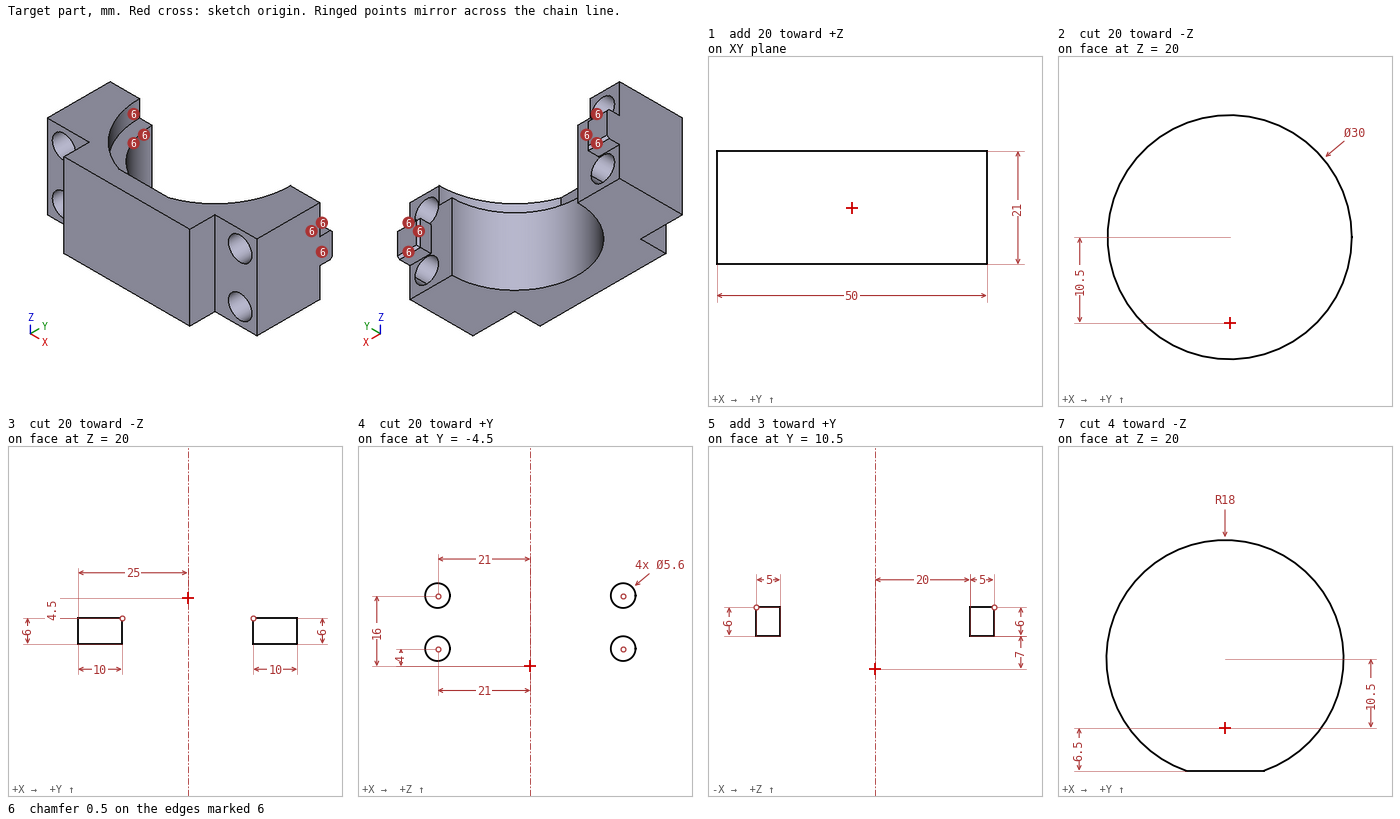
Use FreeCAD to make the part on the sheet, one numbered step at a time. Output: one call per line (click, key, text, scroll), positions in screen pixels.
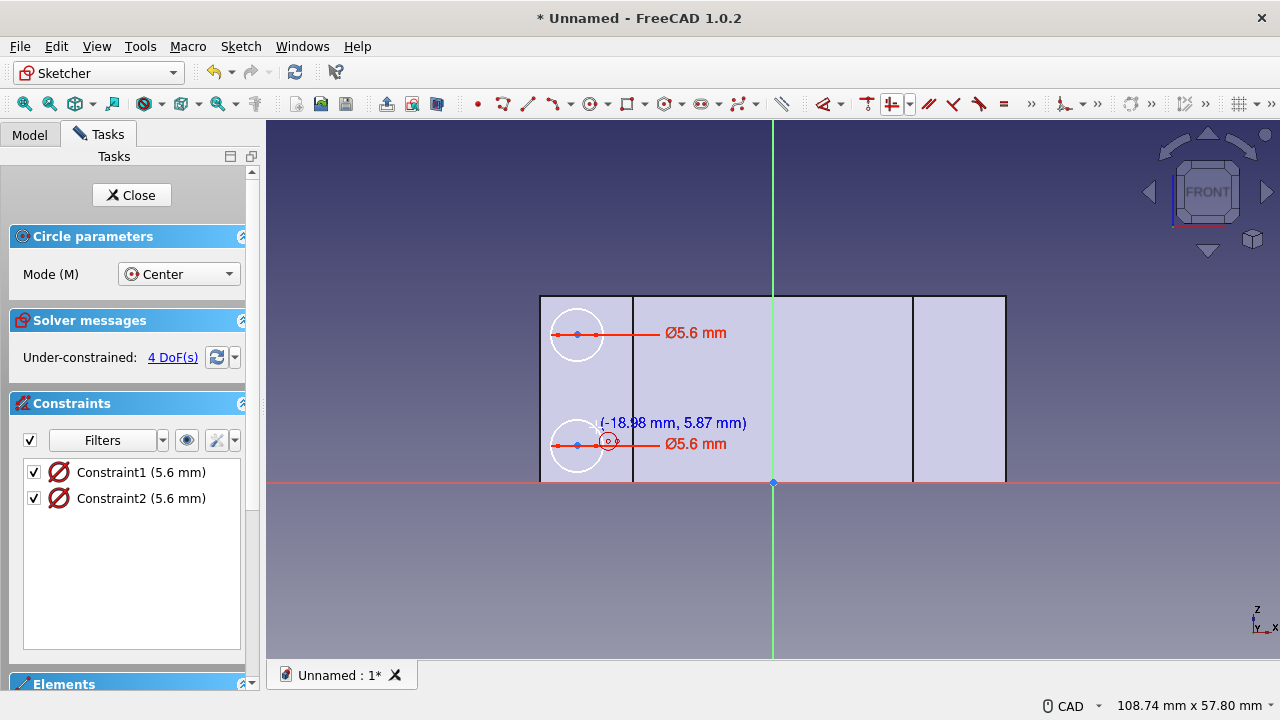
click(969, 334)
move(987, 315)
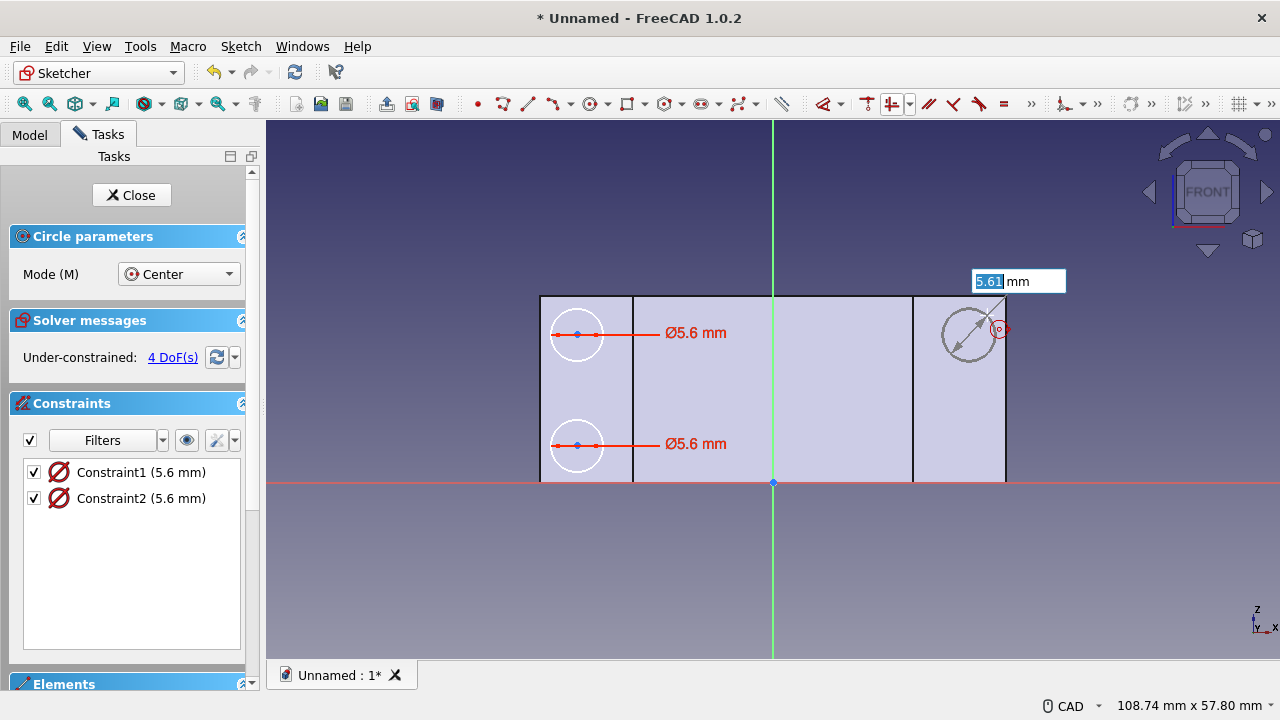
text(5.6)
key(Return)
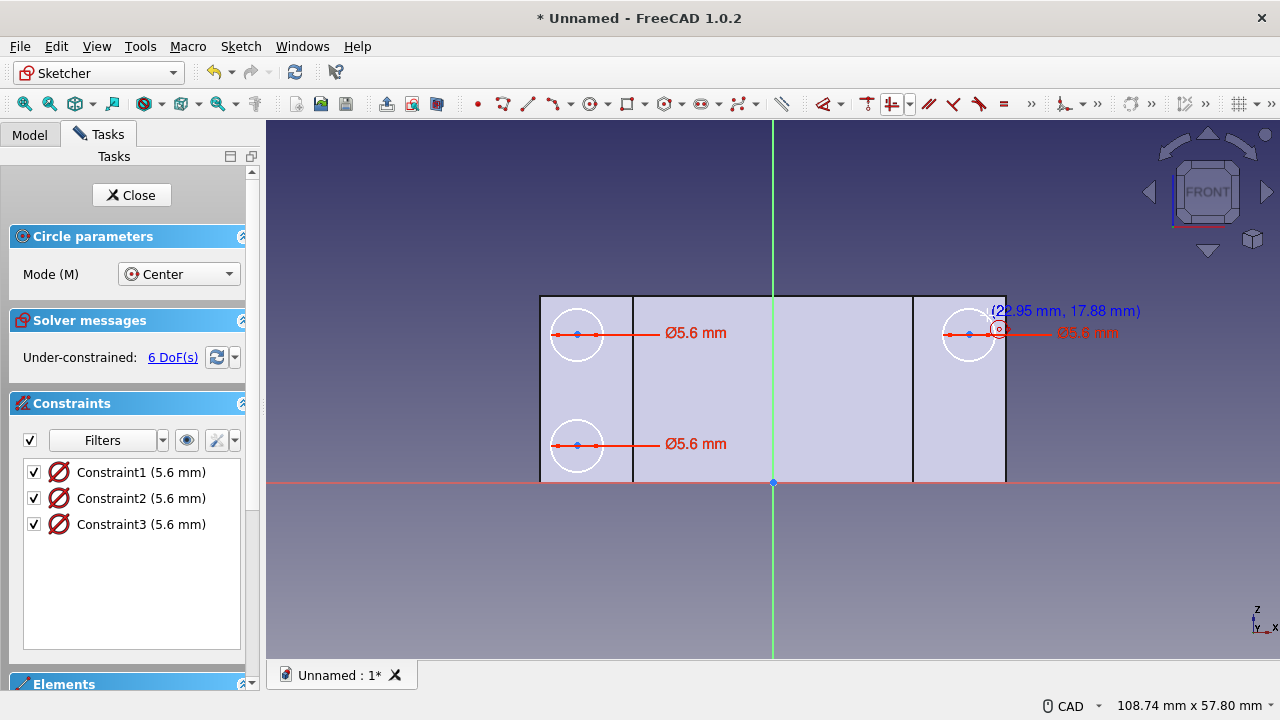
click(969, 445)
move(987, 427)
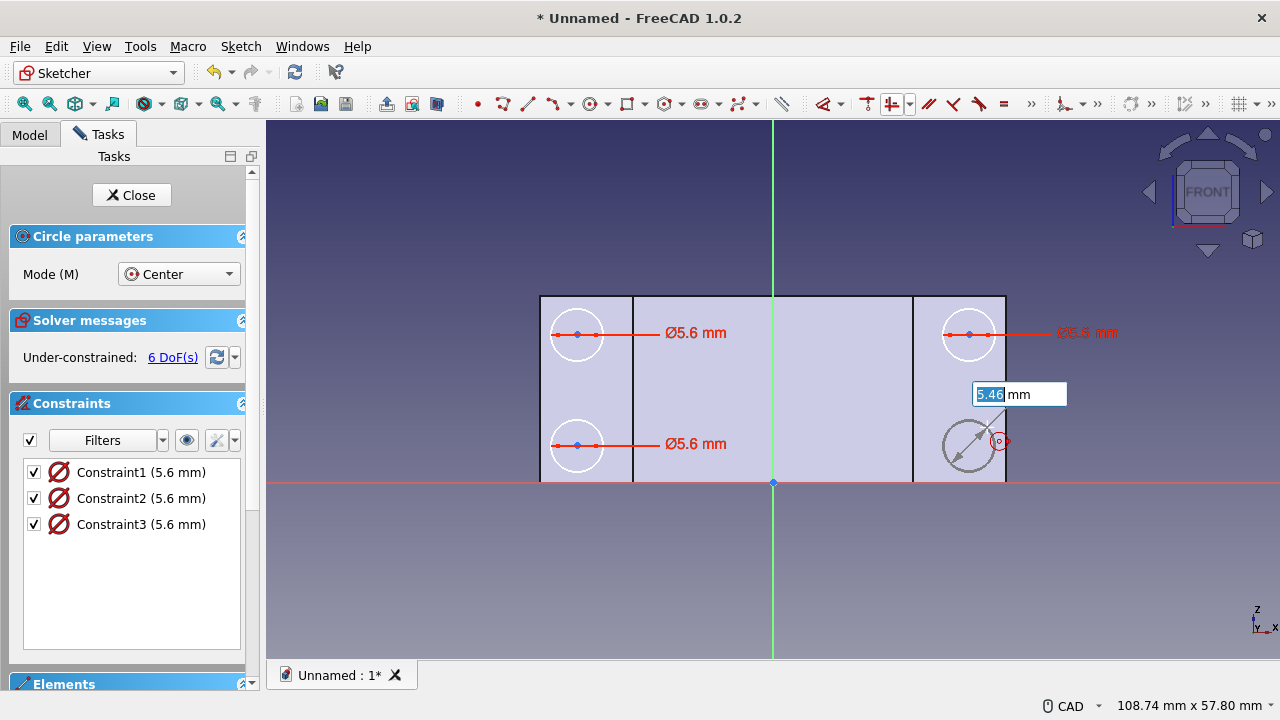
text(5.6)
key(Return)
key(Escape)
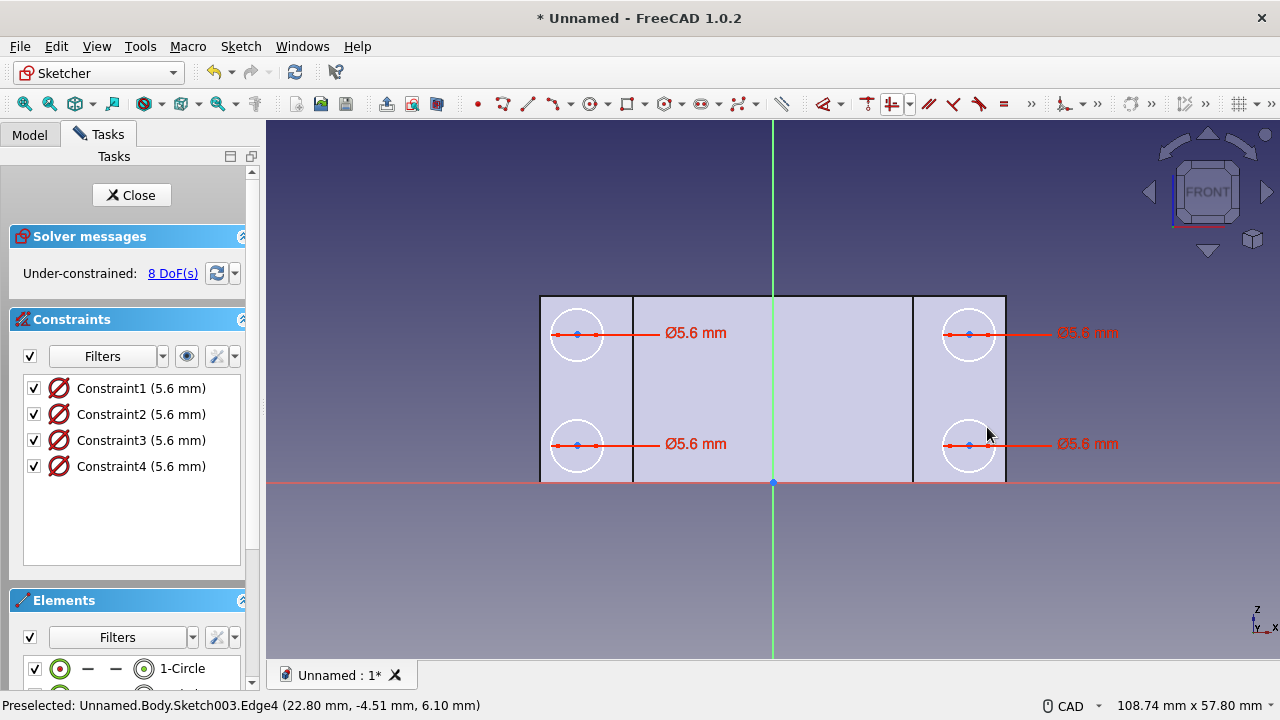
click(577, 335)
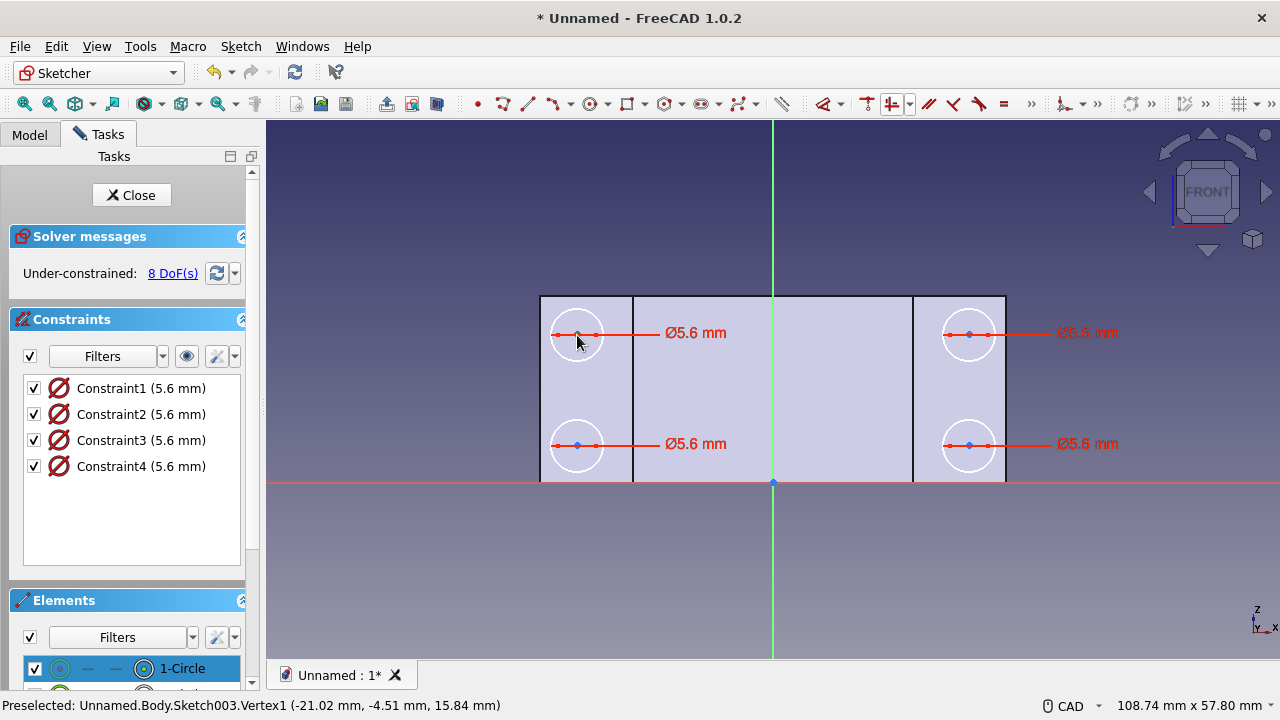
click(969, 335)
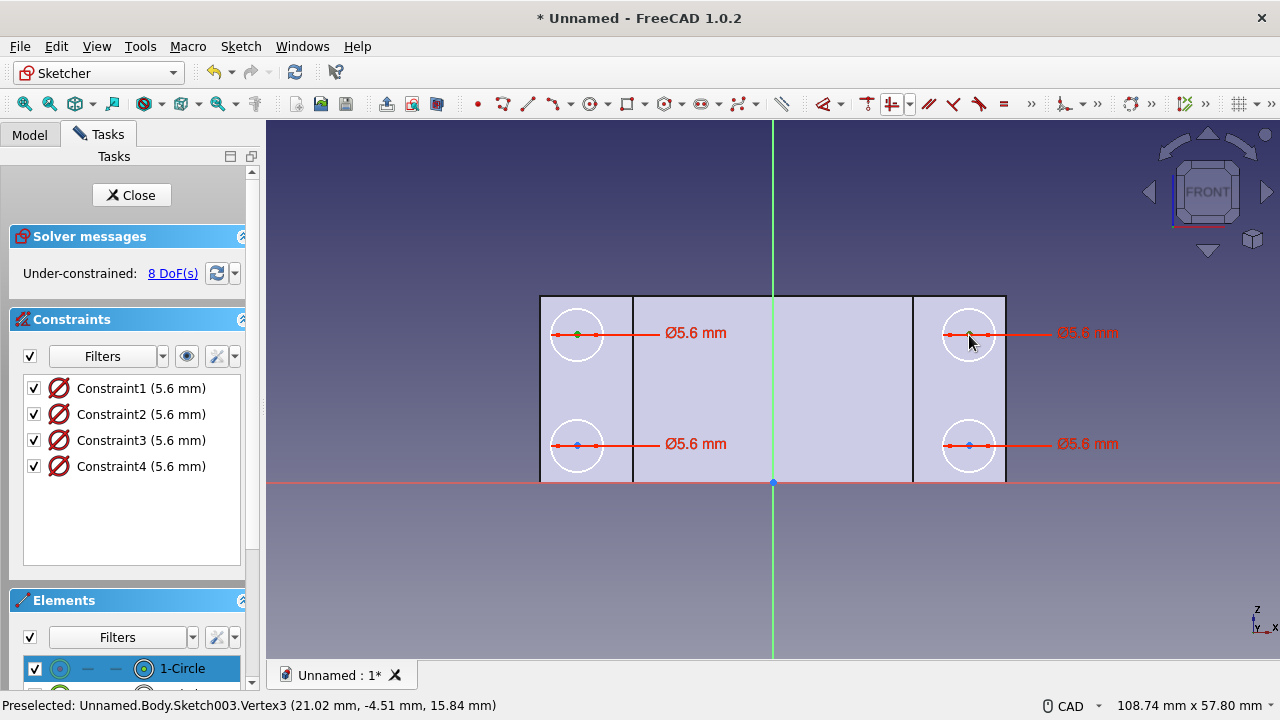
click(773, 596)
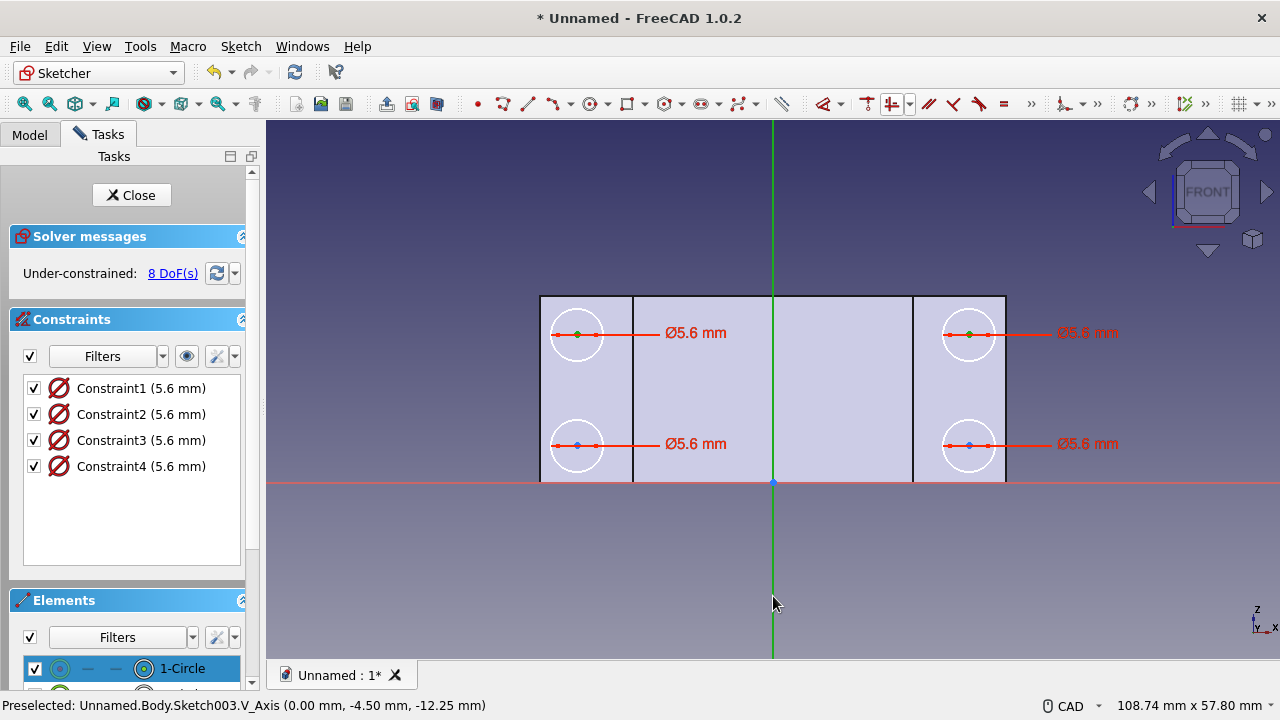
key(s)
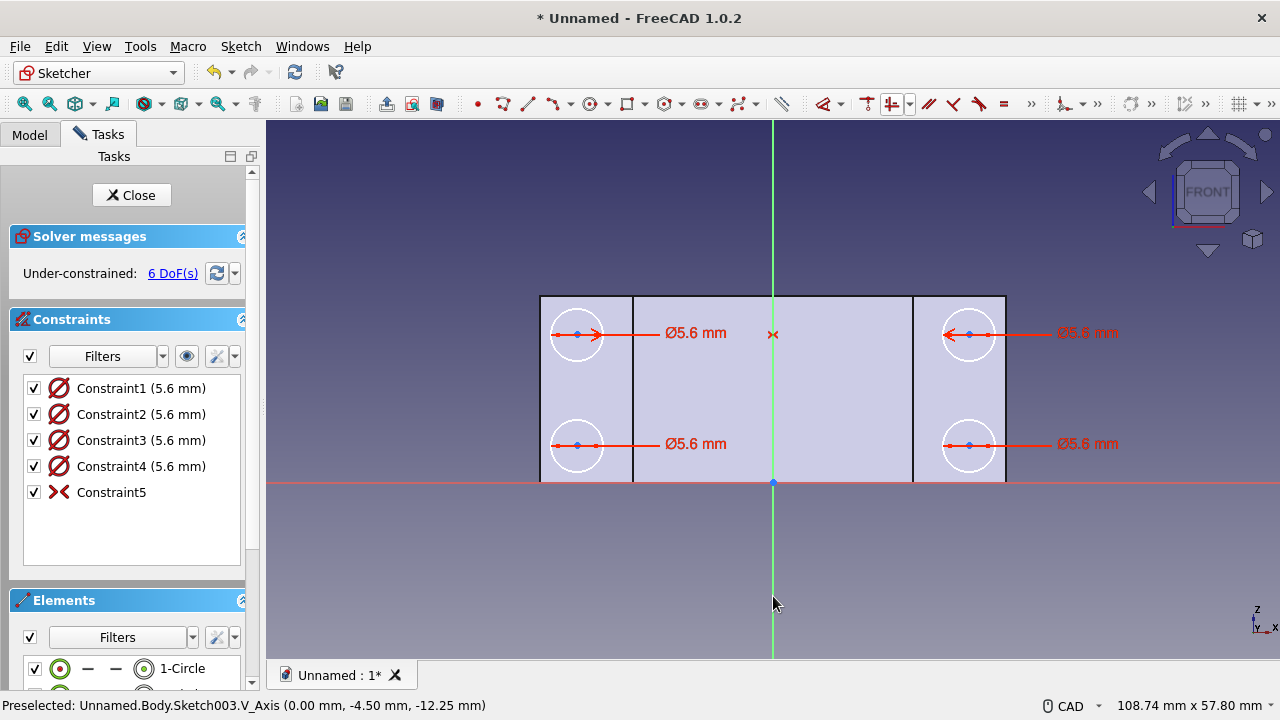
click(577, 446)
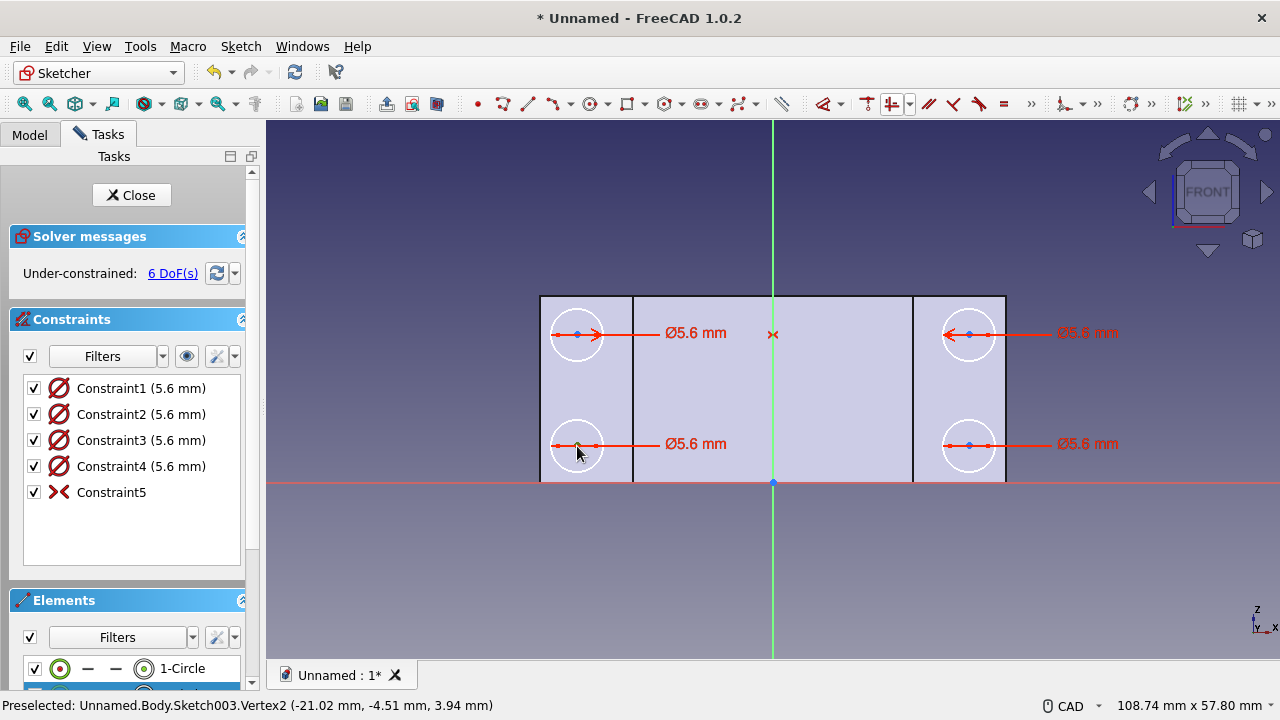
click(969, 446)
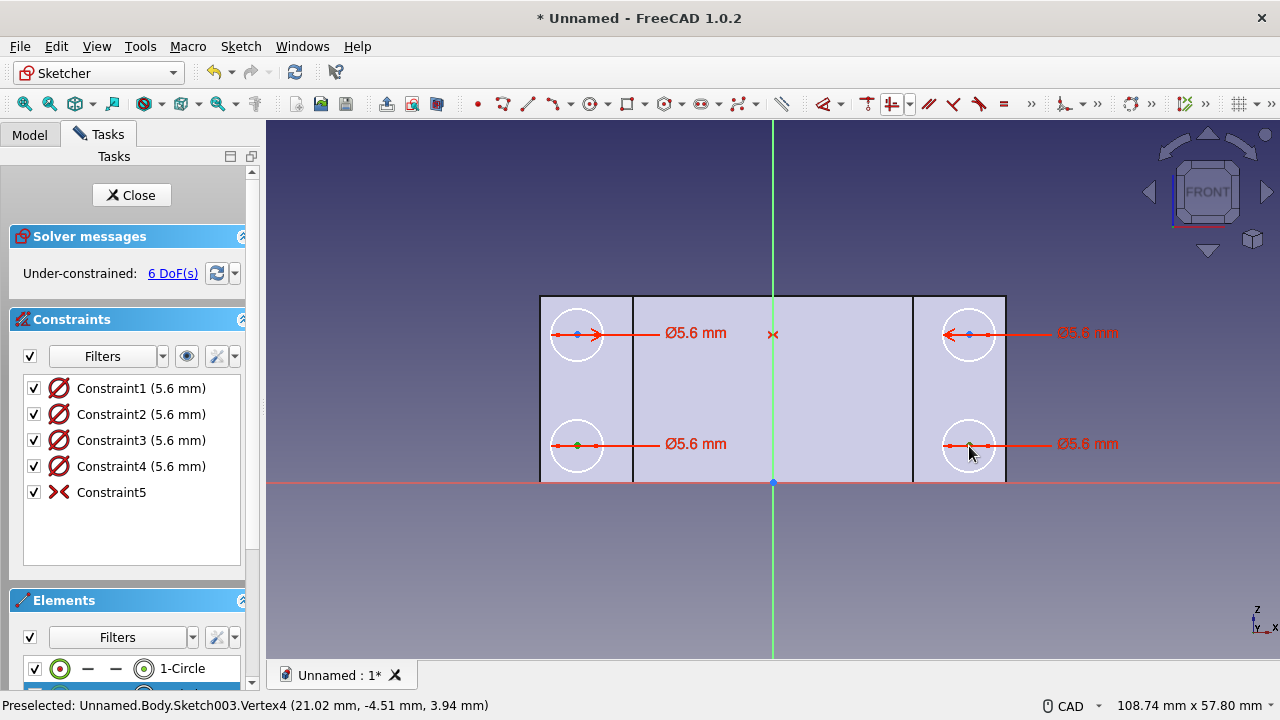
click(773, 596)